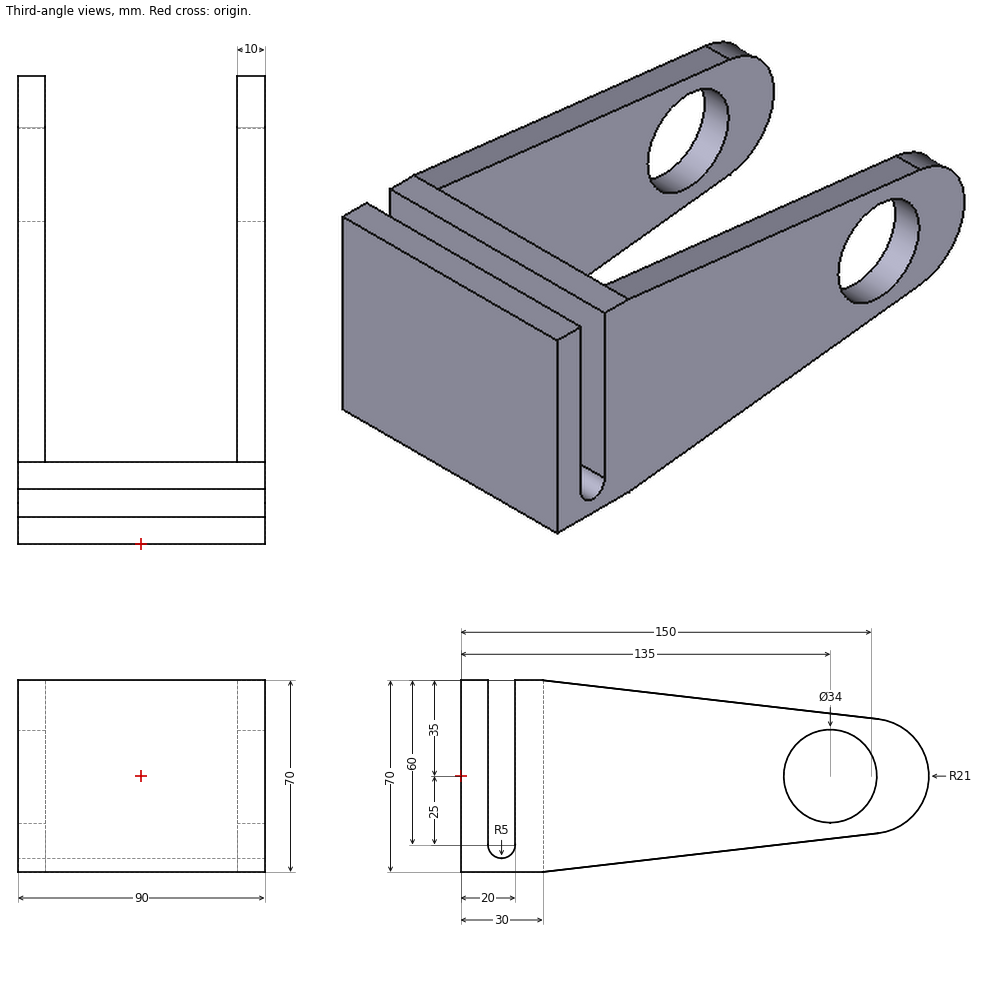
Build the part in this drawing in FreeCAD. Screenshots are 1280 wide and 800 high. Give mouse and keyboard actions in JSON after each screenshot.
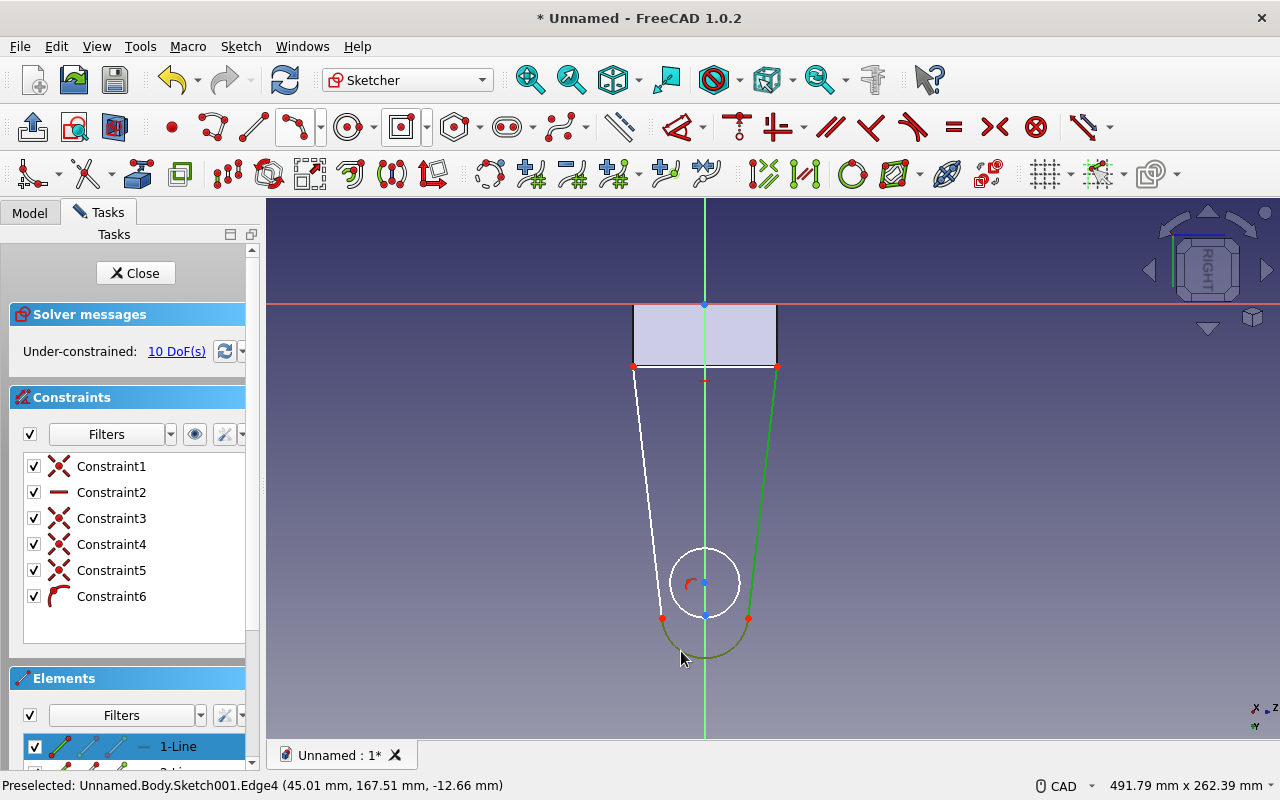
{"action": "left_click", "coordinate": [913, 128]}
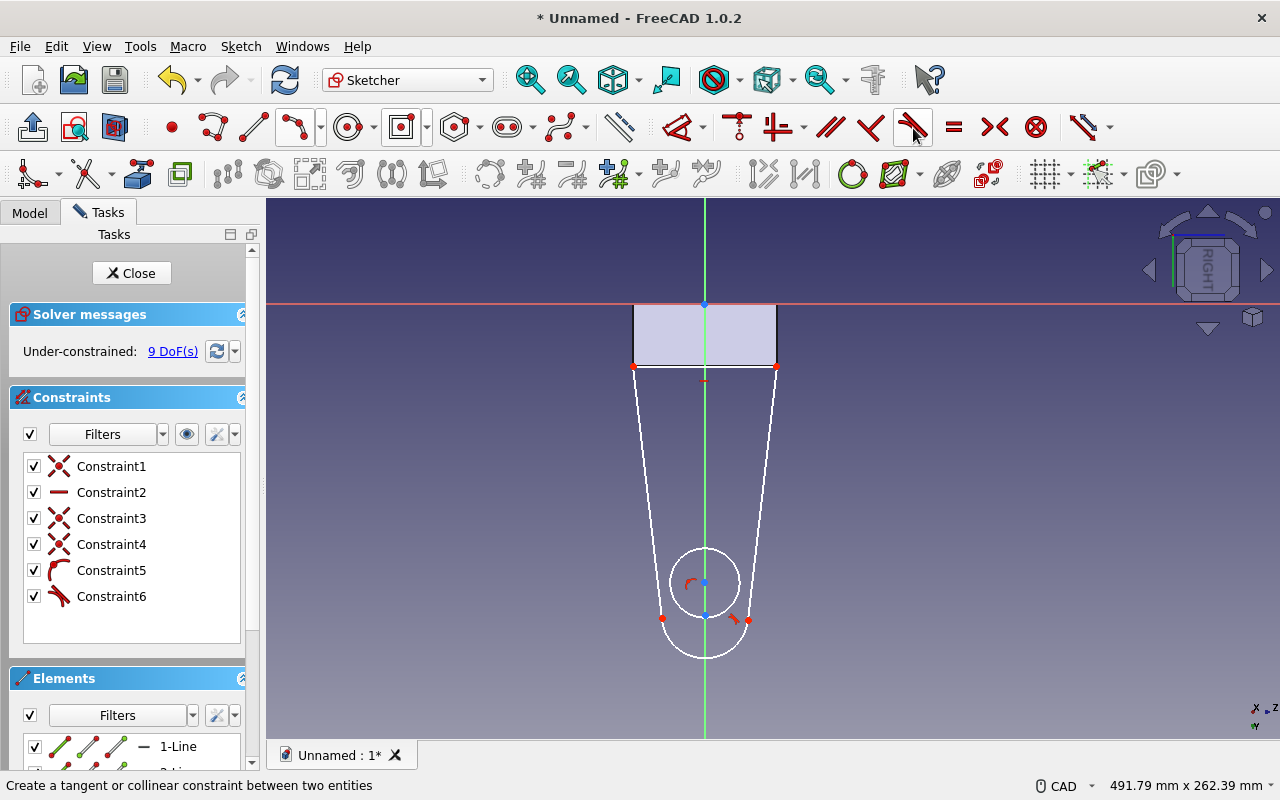
{"action": "left_click", "coordinate": [642, 443]}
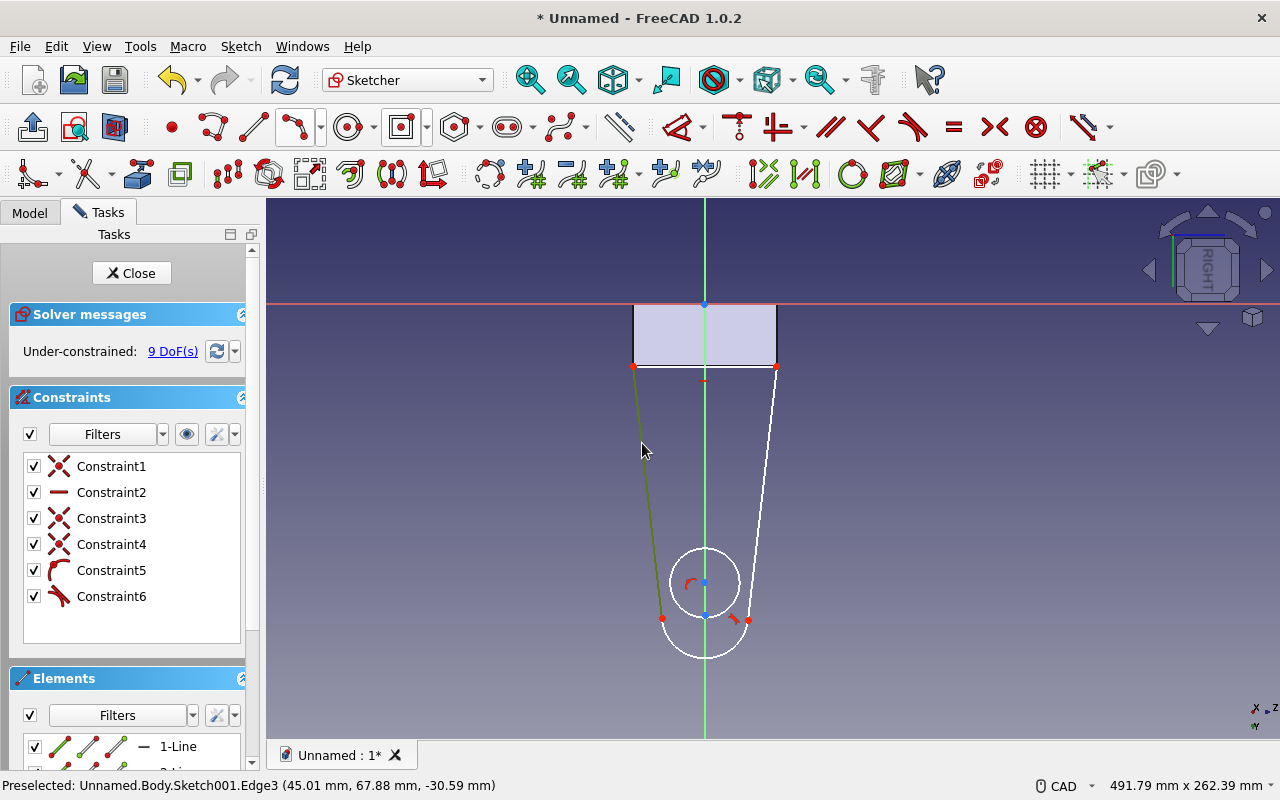
{"action": "left_click", "coordinate": [681, 651]}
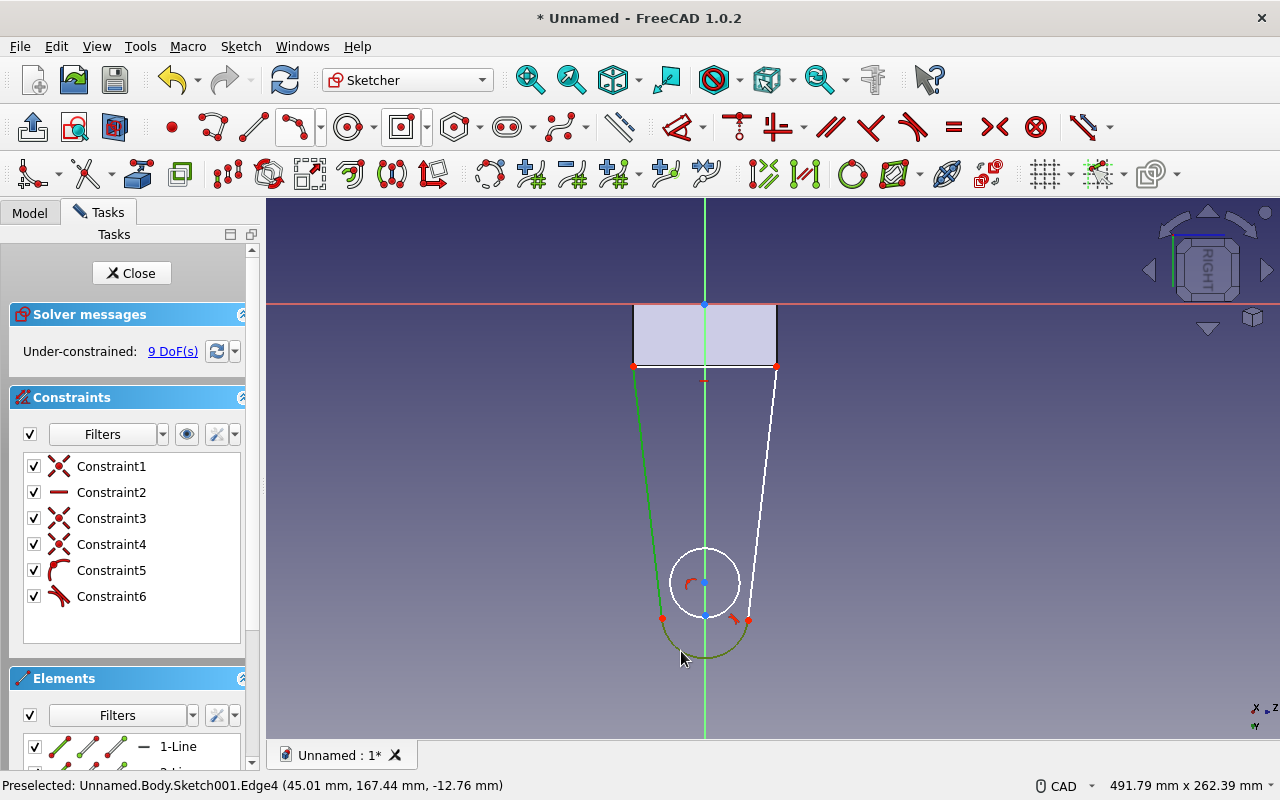
{"action": "left_click", "coordinate": [913, 128]}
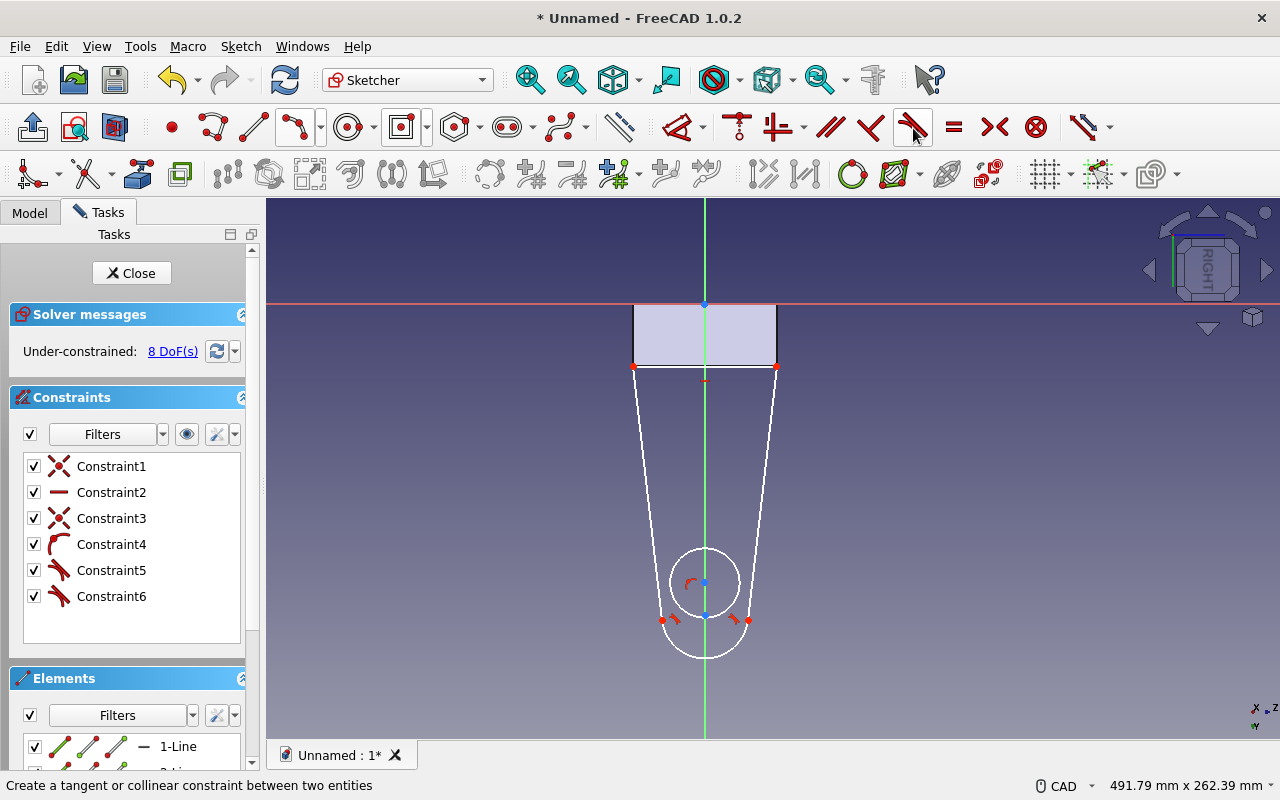
{"action": "left_click", "coordinate": [705, 615]}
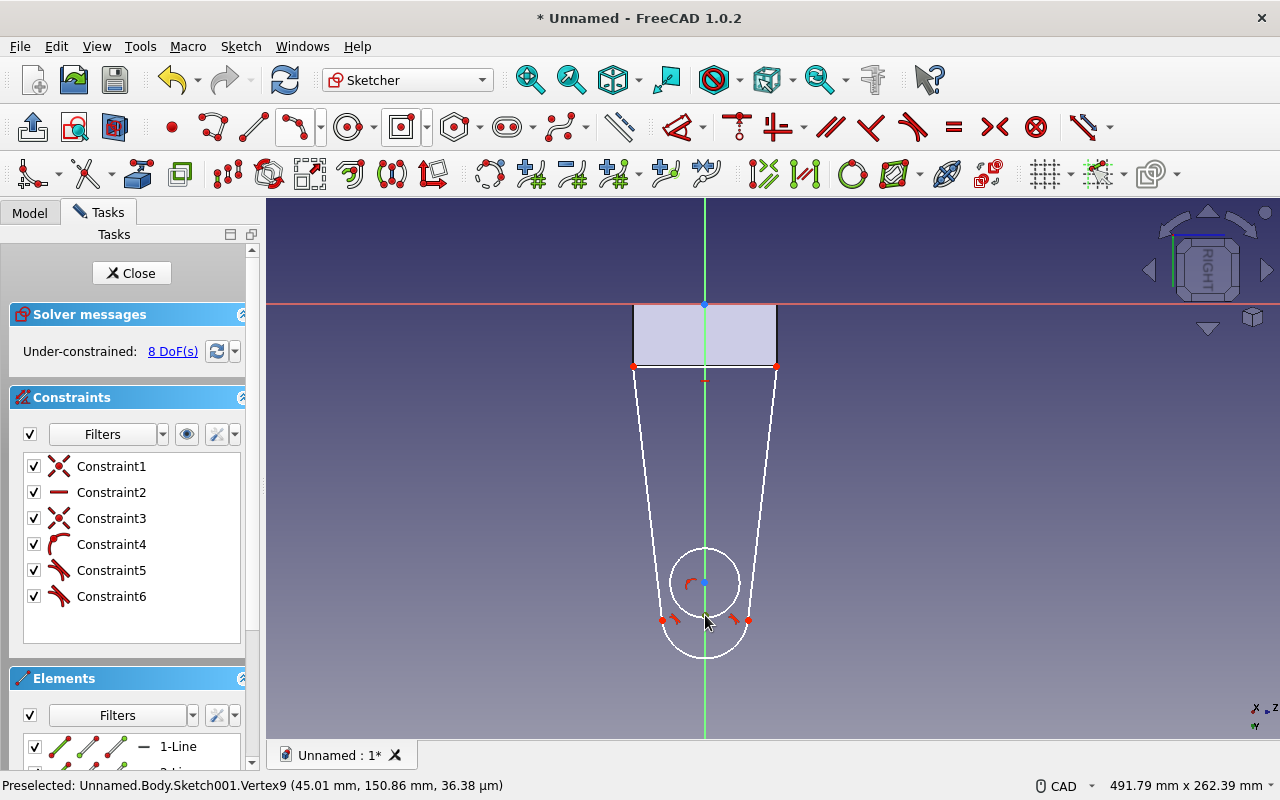
{"action": "left_click", "coordinate": [705, 503]}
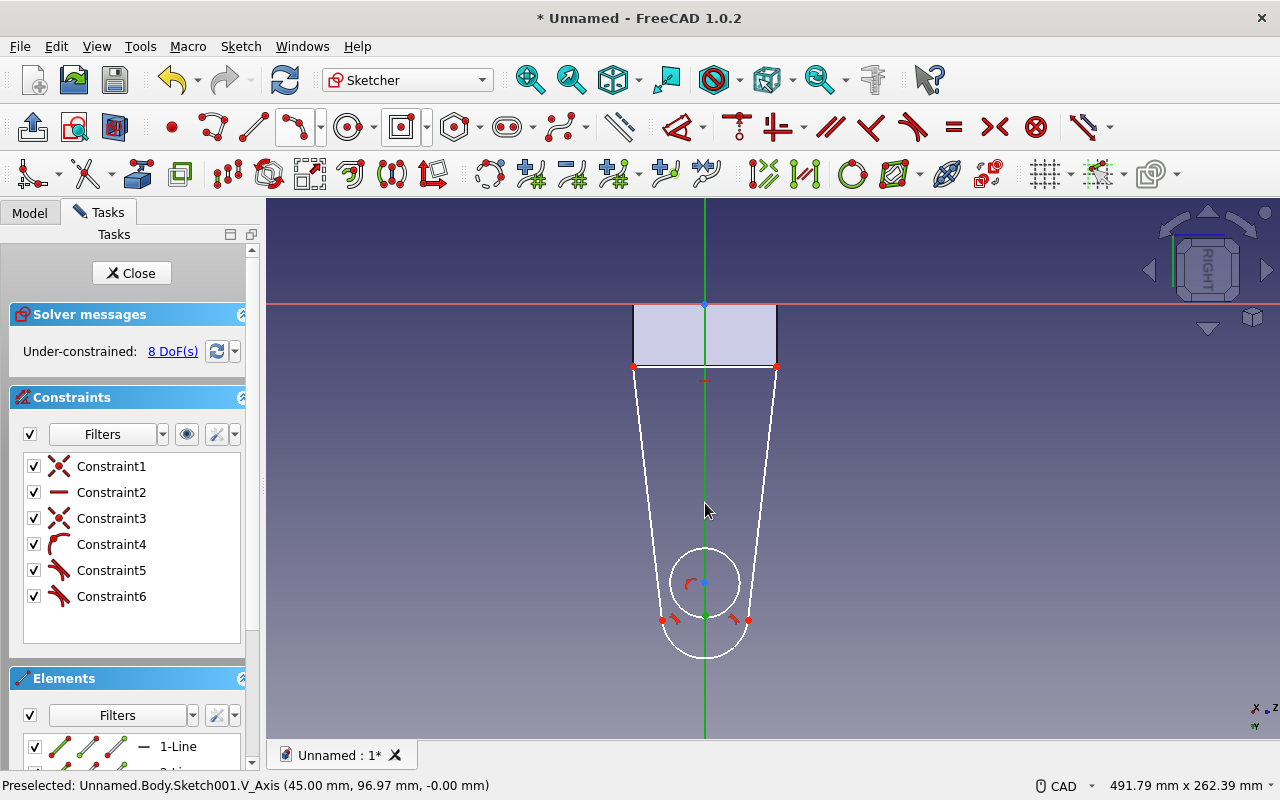
{"action": "left_click", "coordinate": [737, 128]}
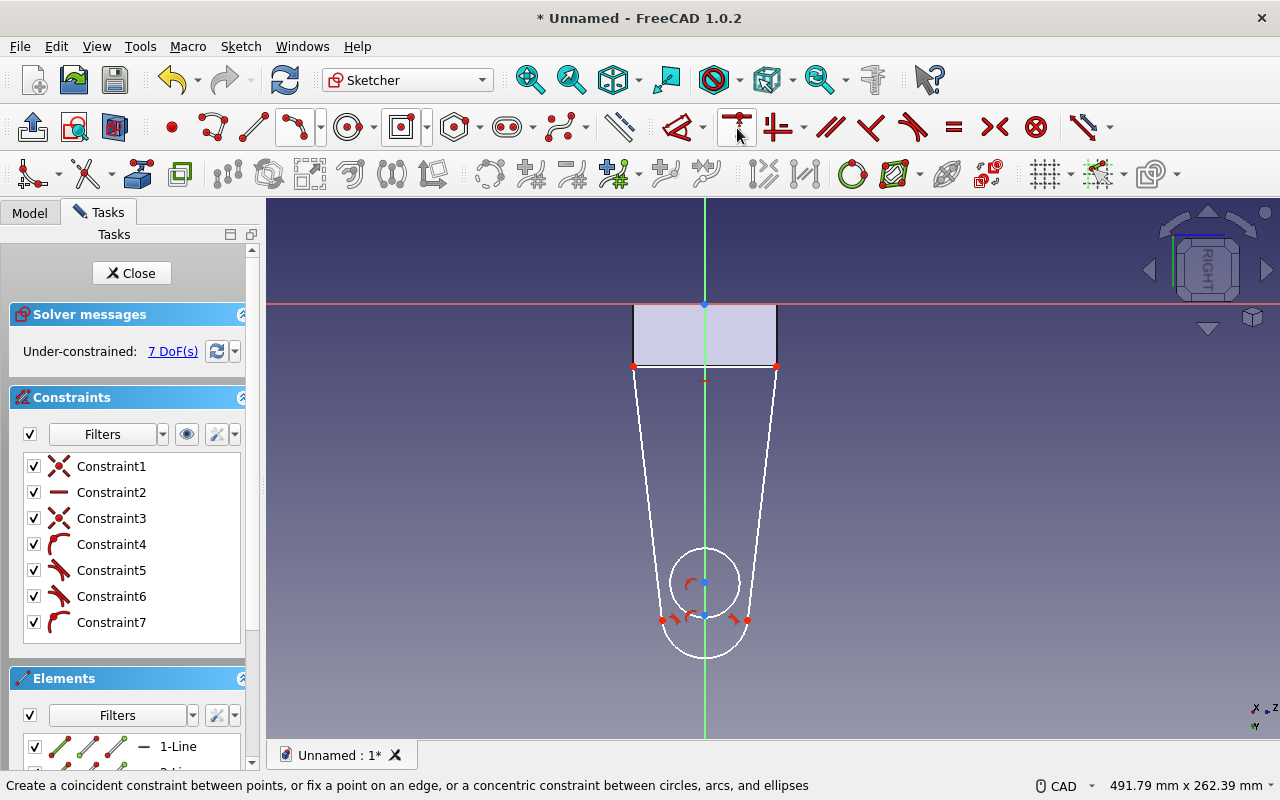
{"action": "left_click", "coordinate": [676, 128]}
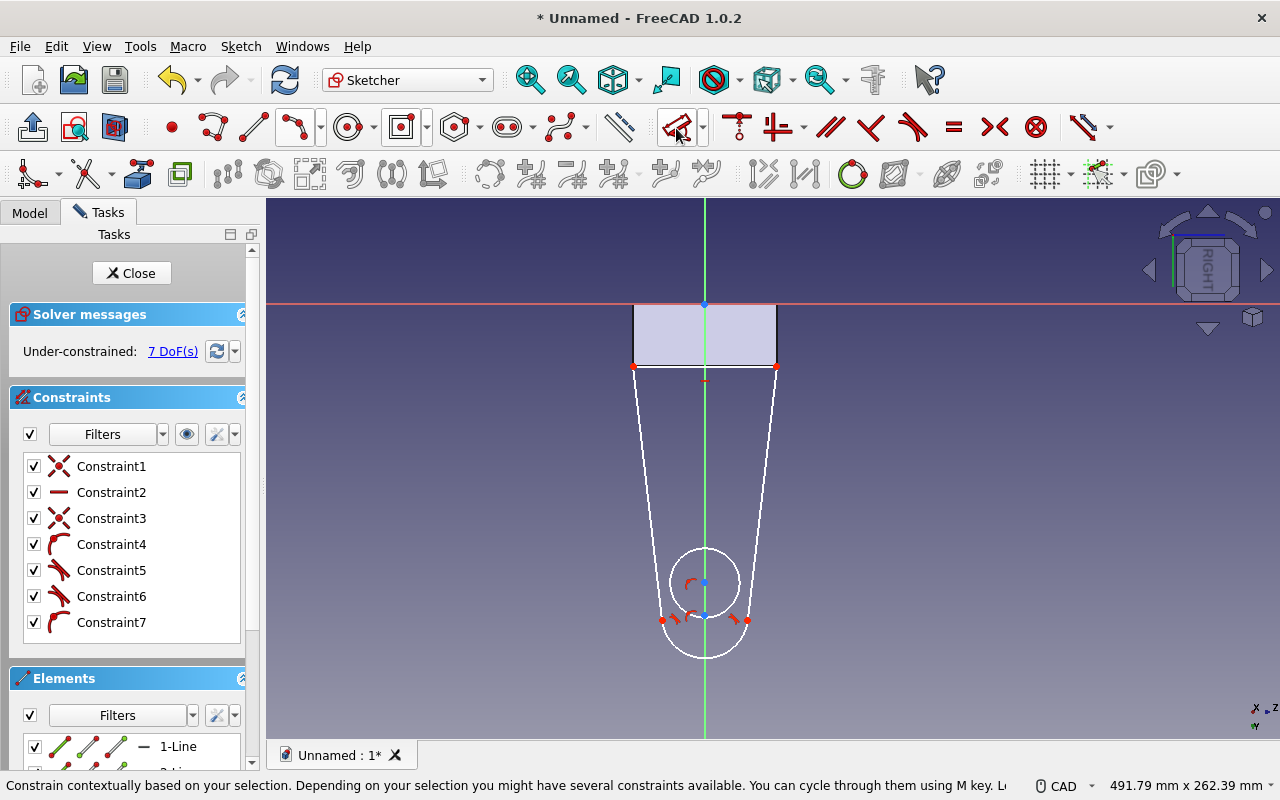
{"action": "left_click", "coordinate": [681, 651]}
{"action": "left_click", "coordinate": [663, 678]}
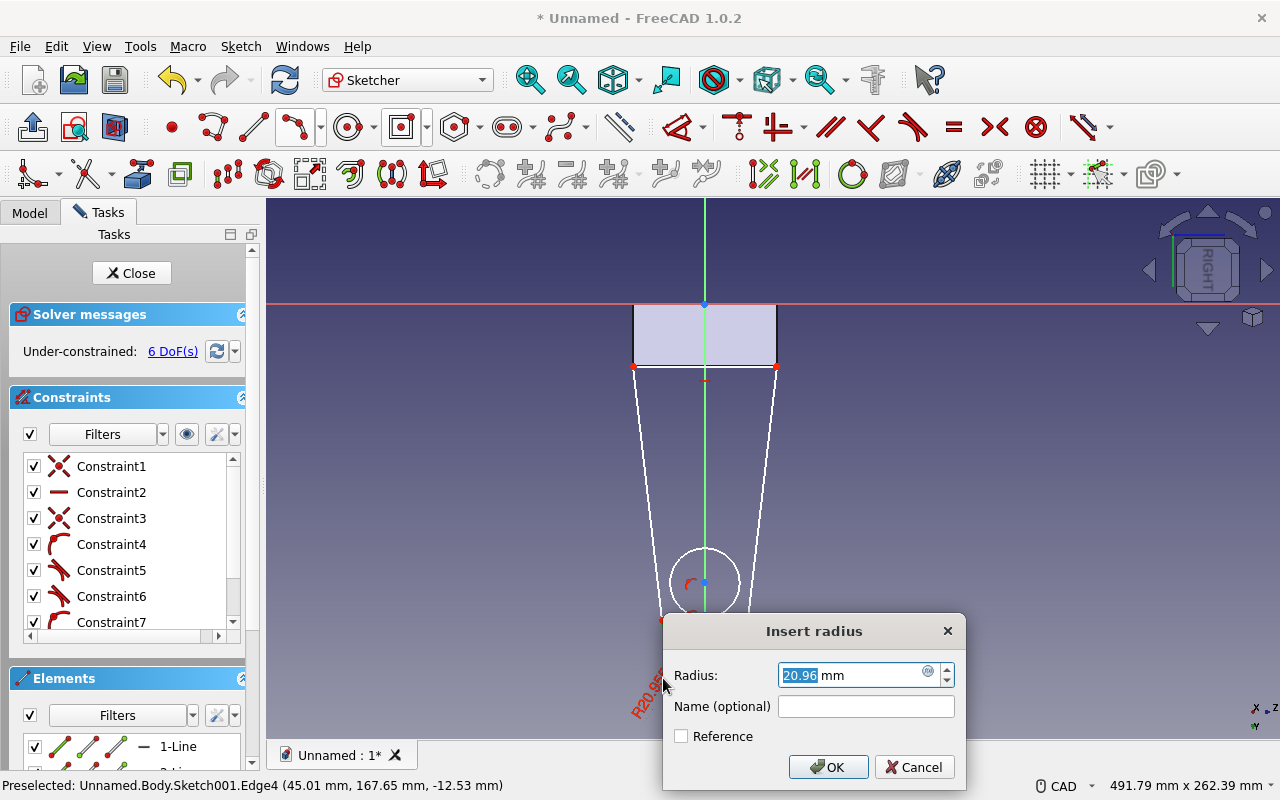
{"action": "type", "text": "21"}
{"action": "key", "text": "Return"}